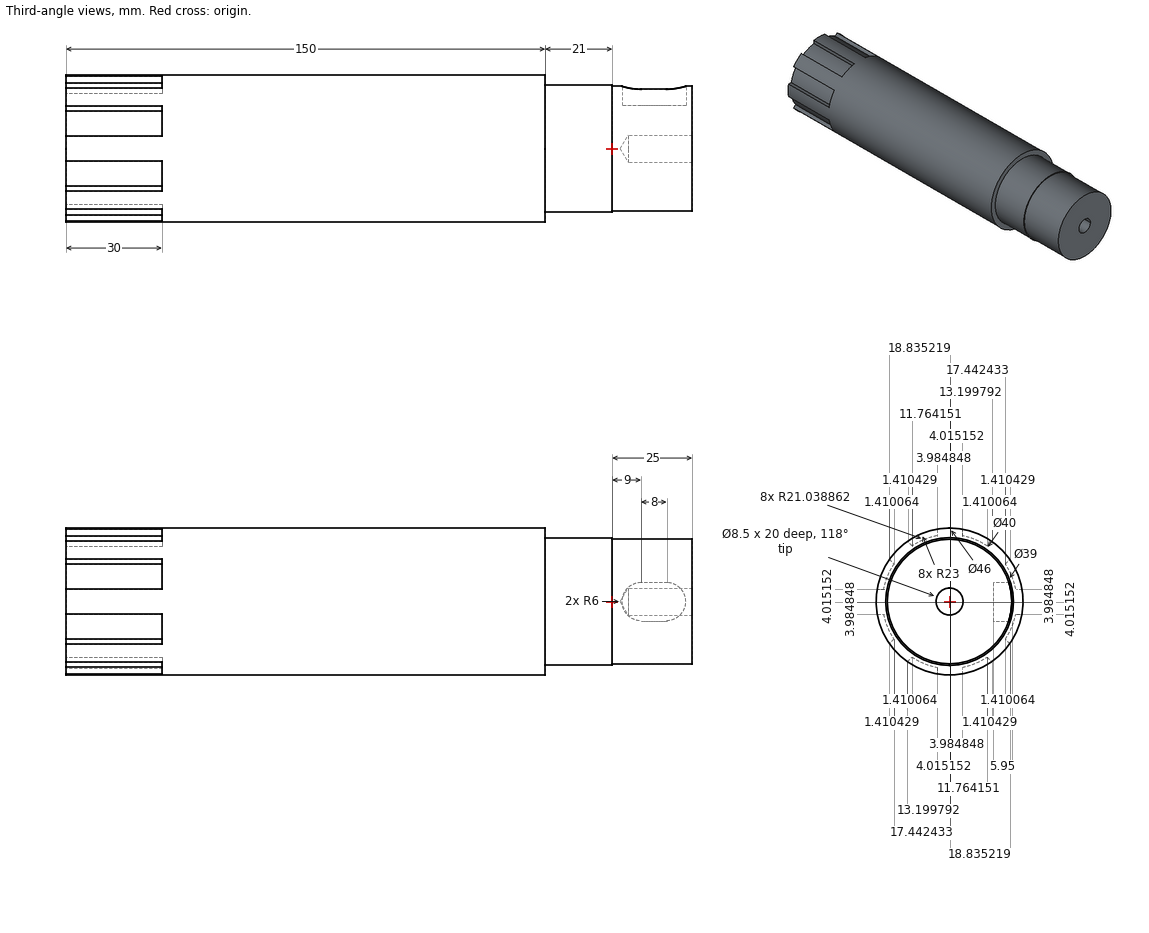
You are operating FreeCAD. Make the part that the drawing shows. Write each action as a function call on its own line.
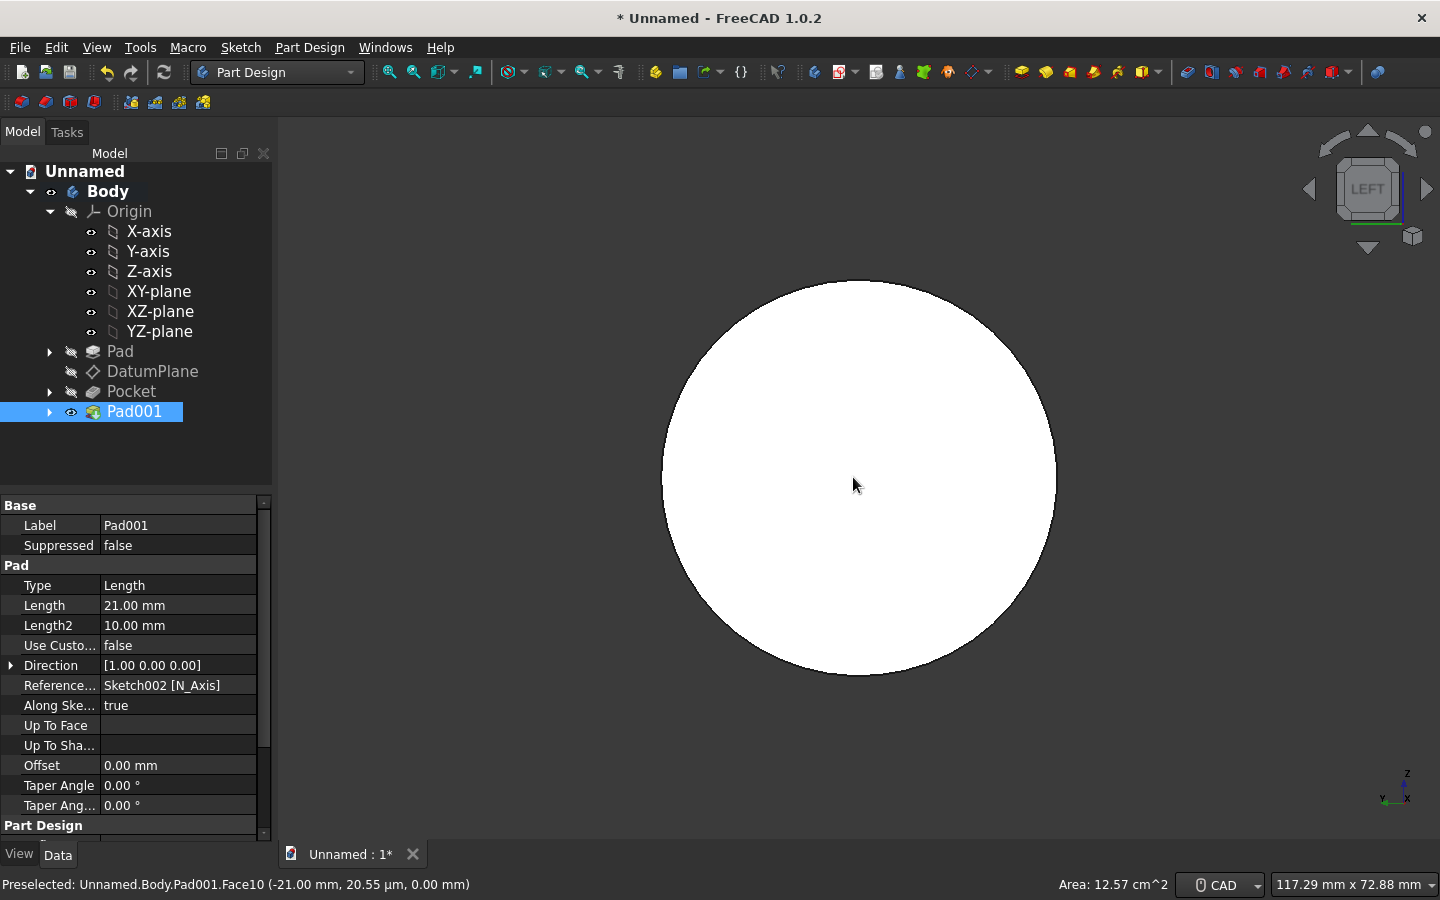
click(840, 72)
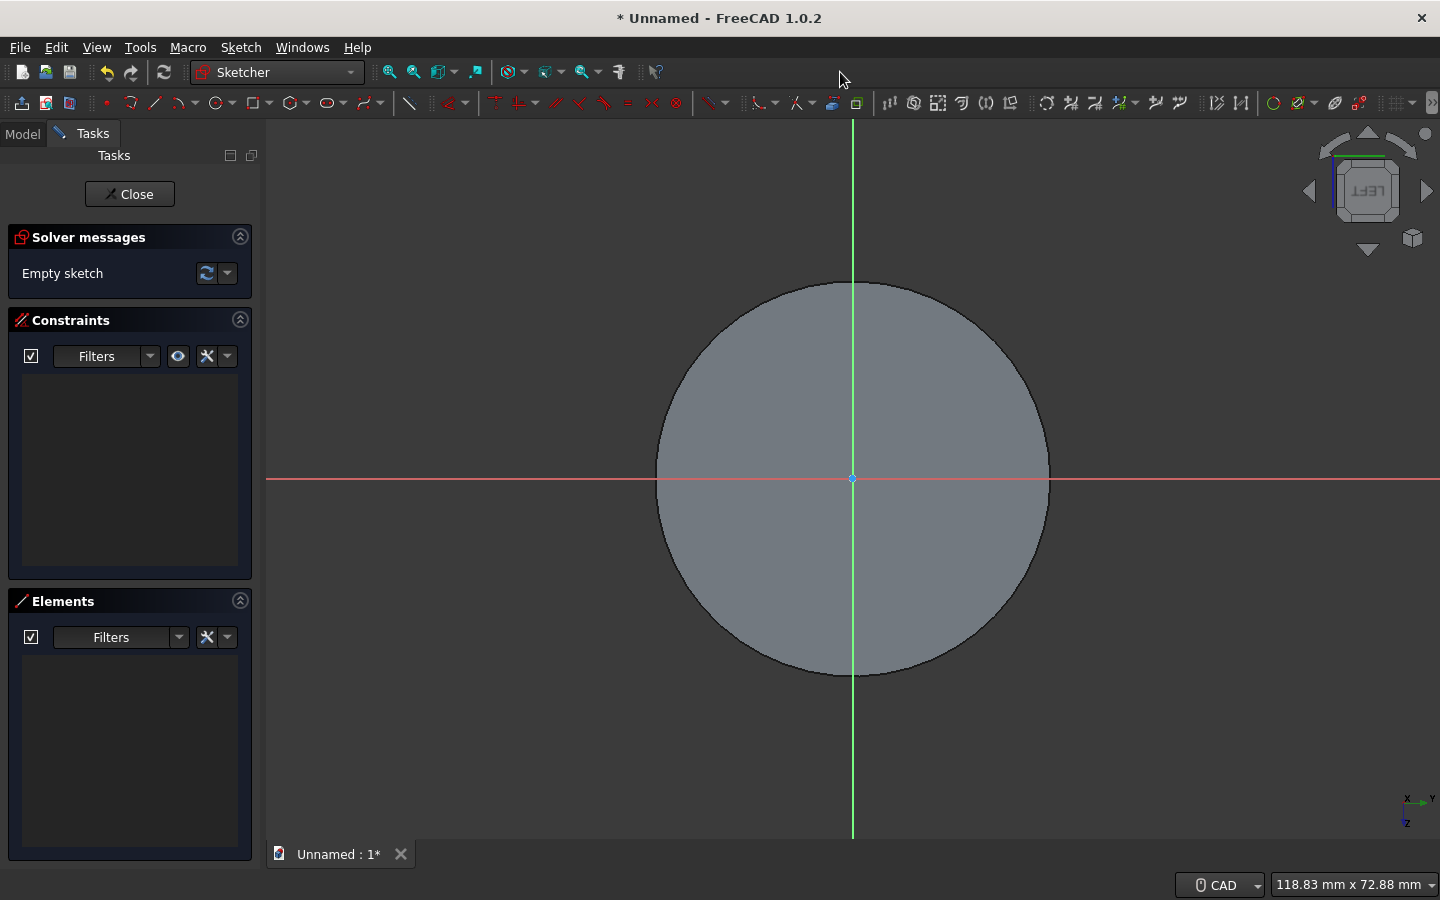
click(216, 104)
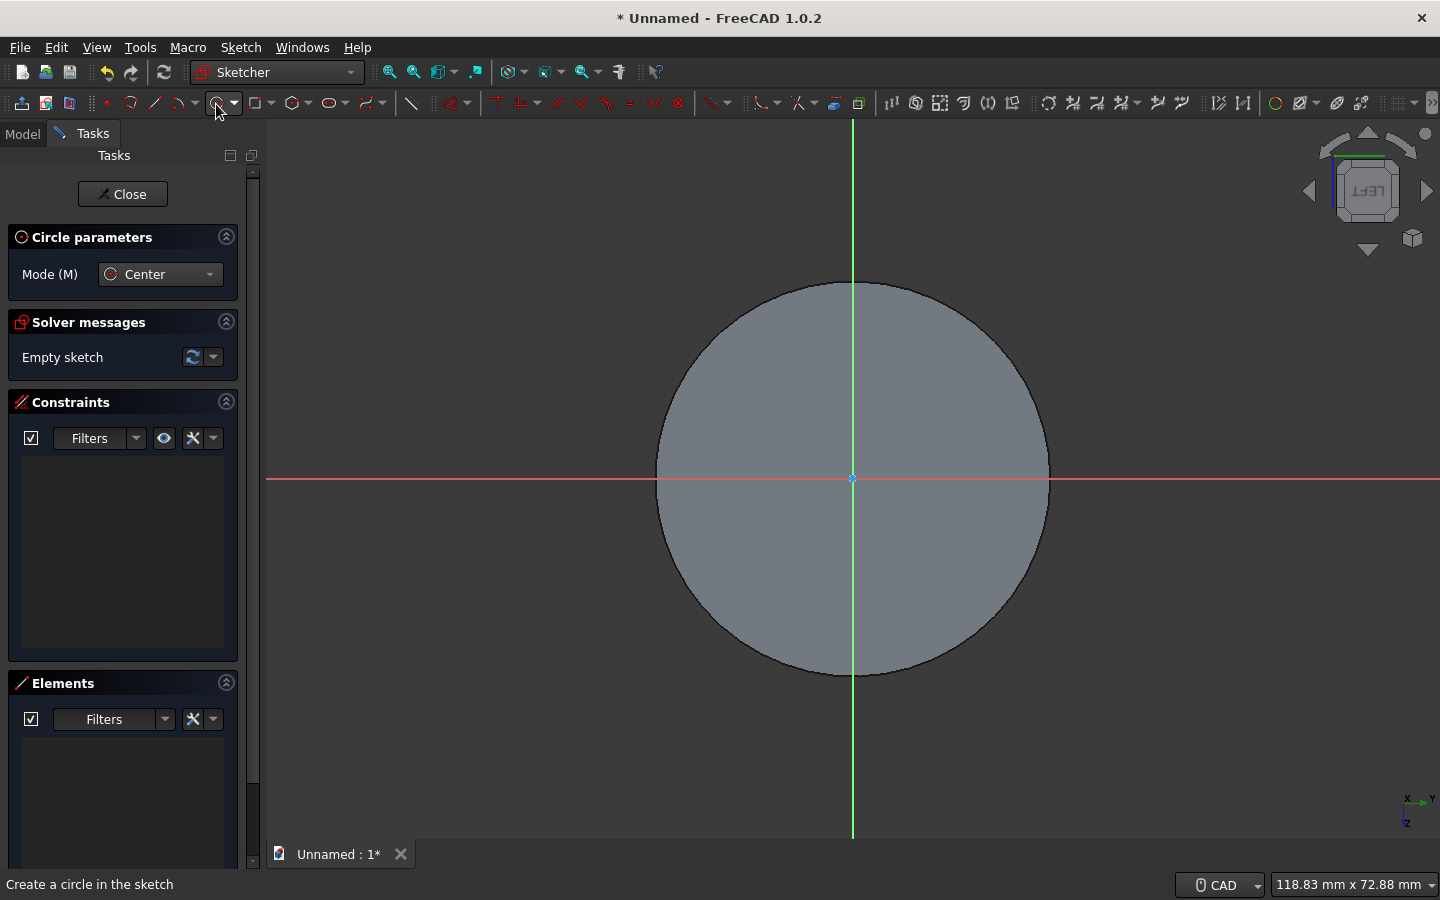
click(853, 479)
click(1013, 318)
key(Escape)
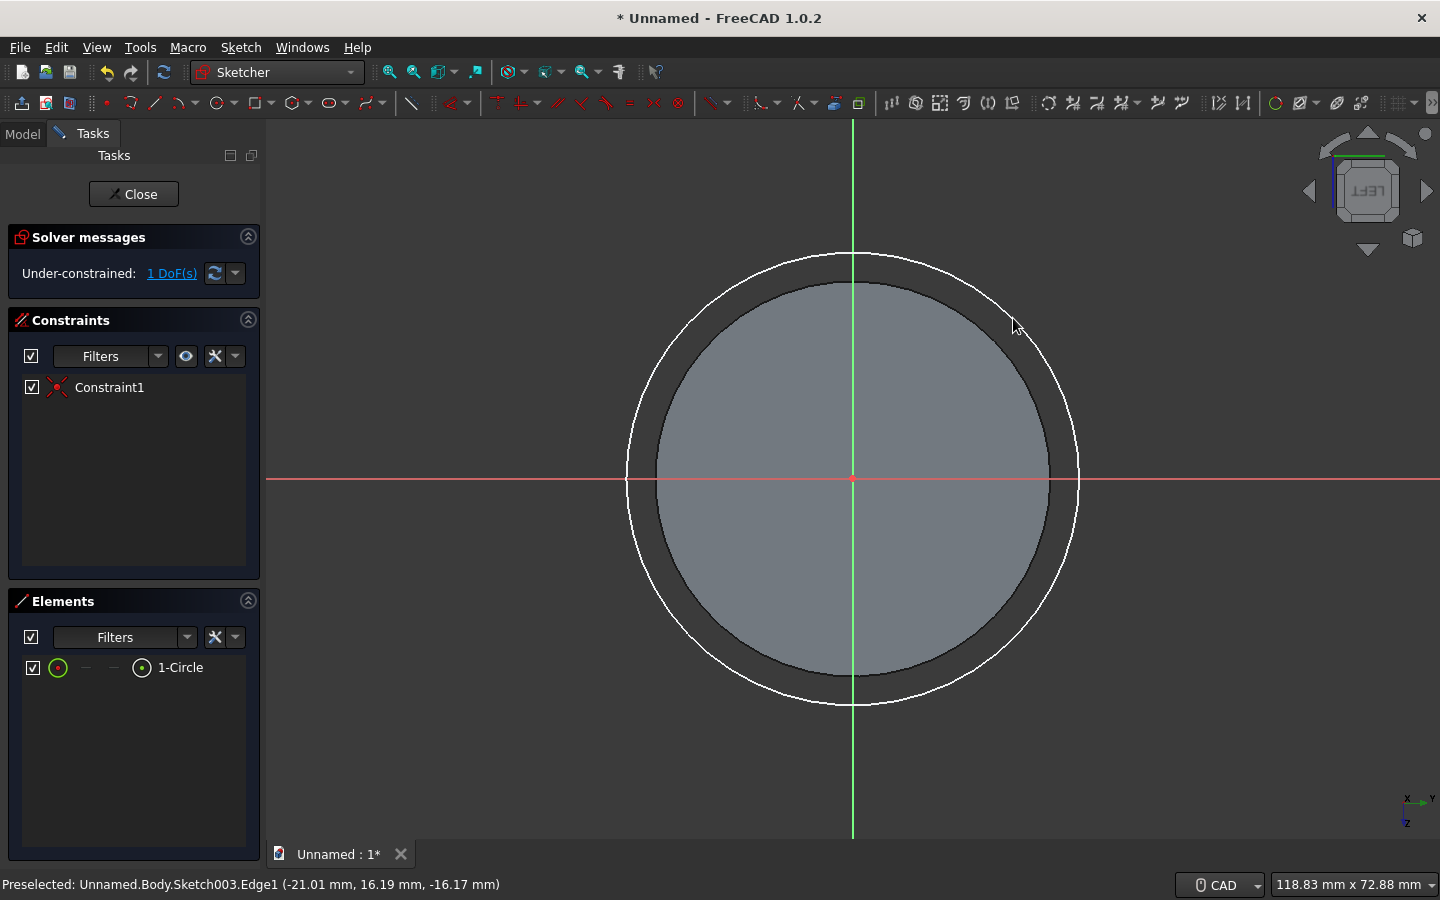
click(450, 104)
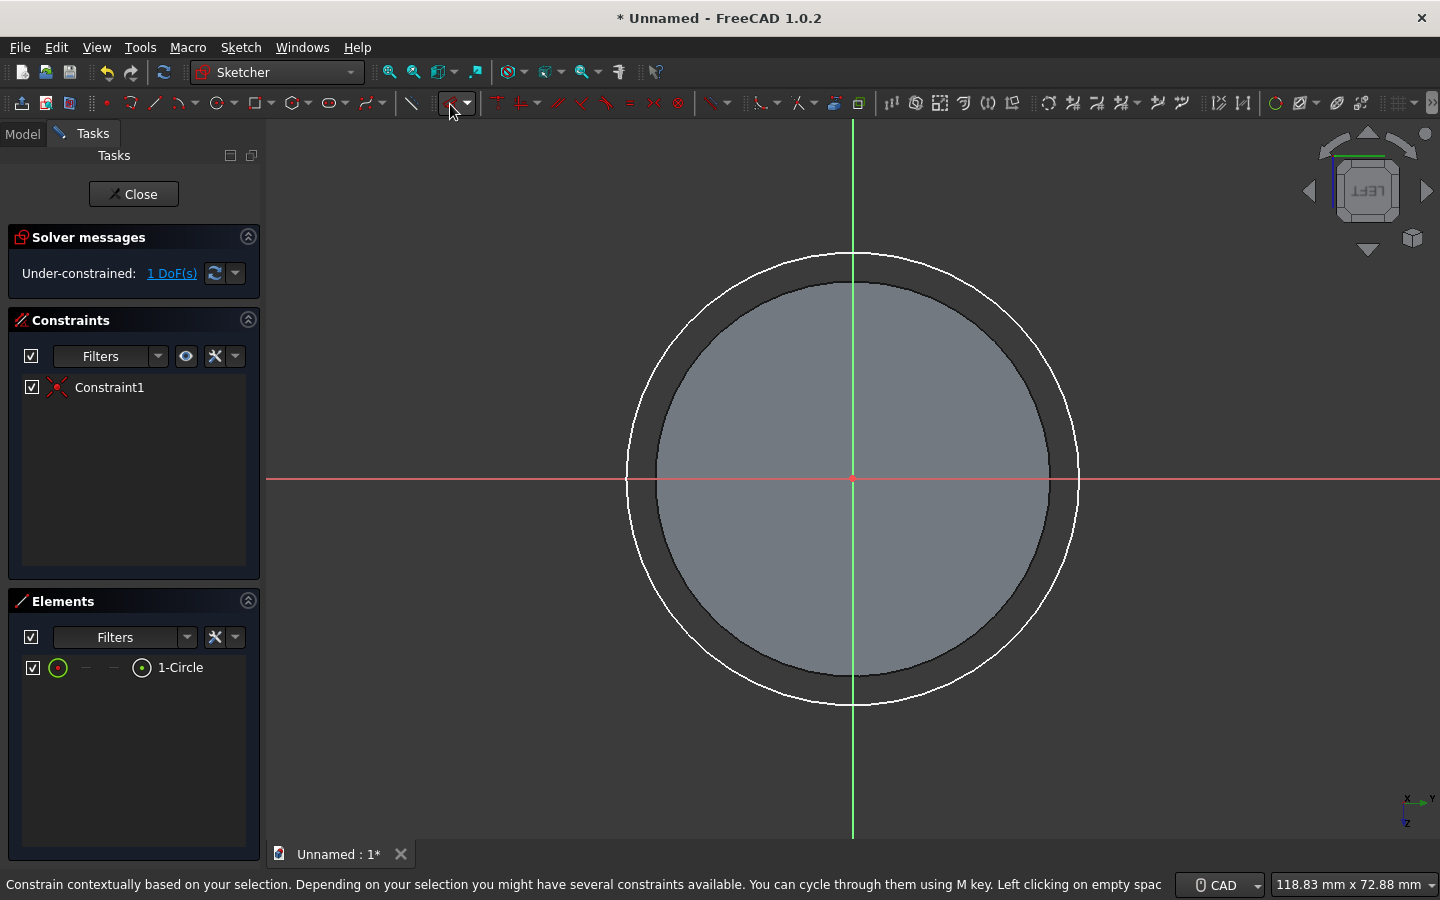
click(1012, 318)
click(1035, 295)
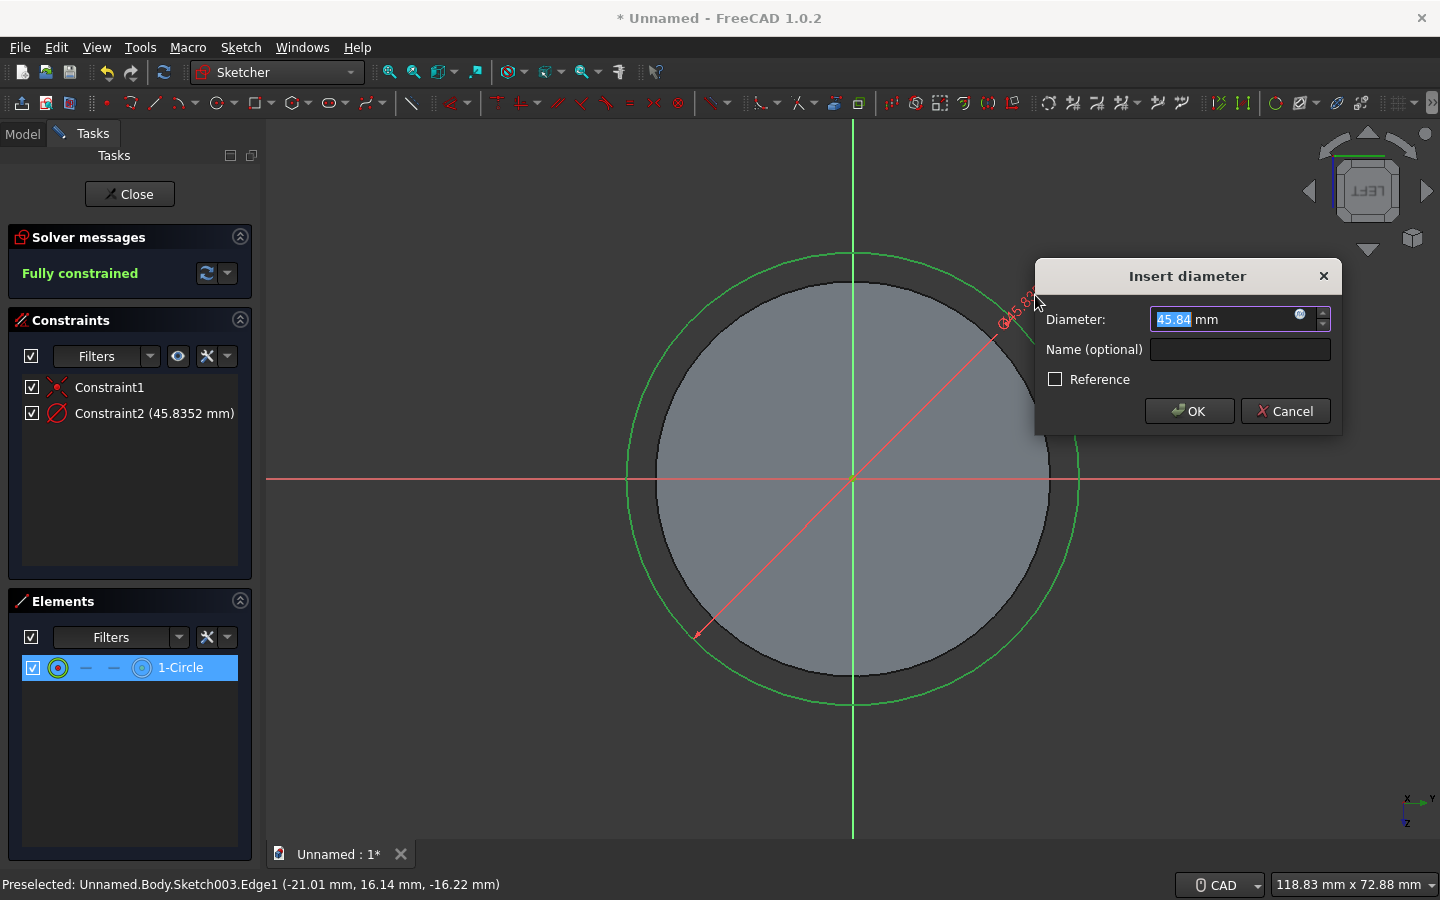
text(46)
key(Return)
key(Escape)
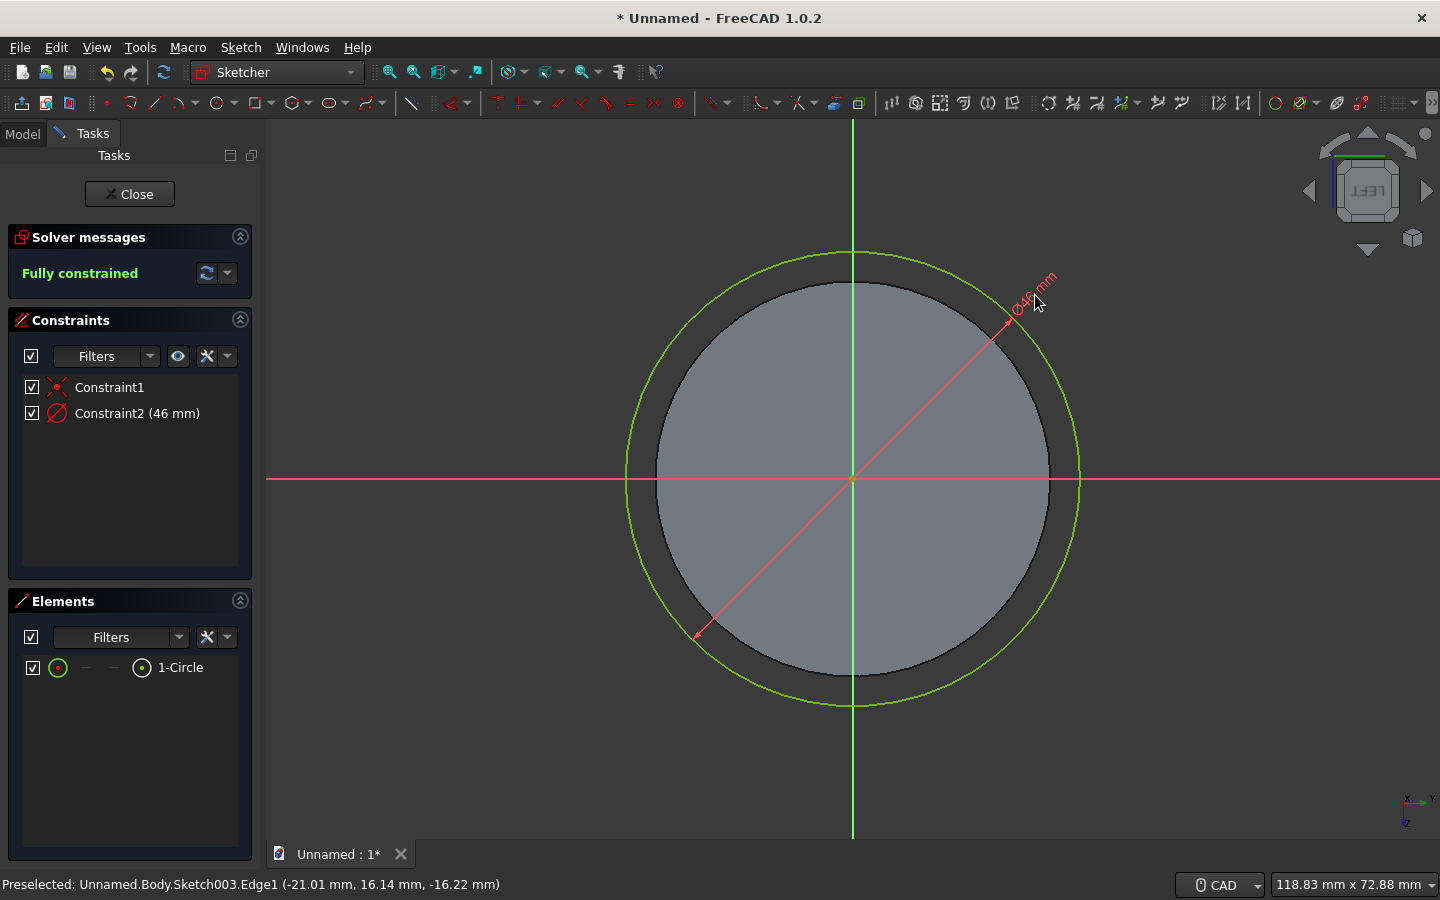
click(130, 194)